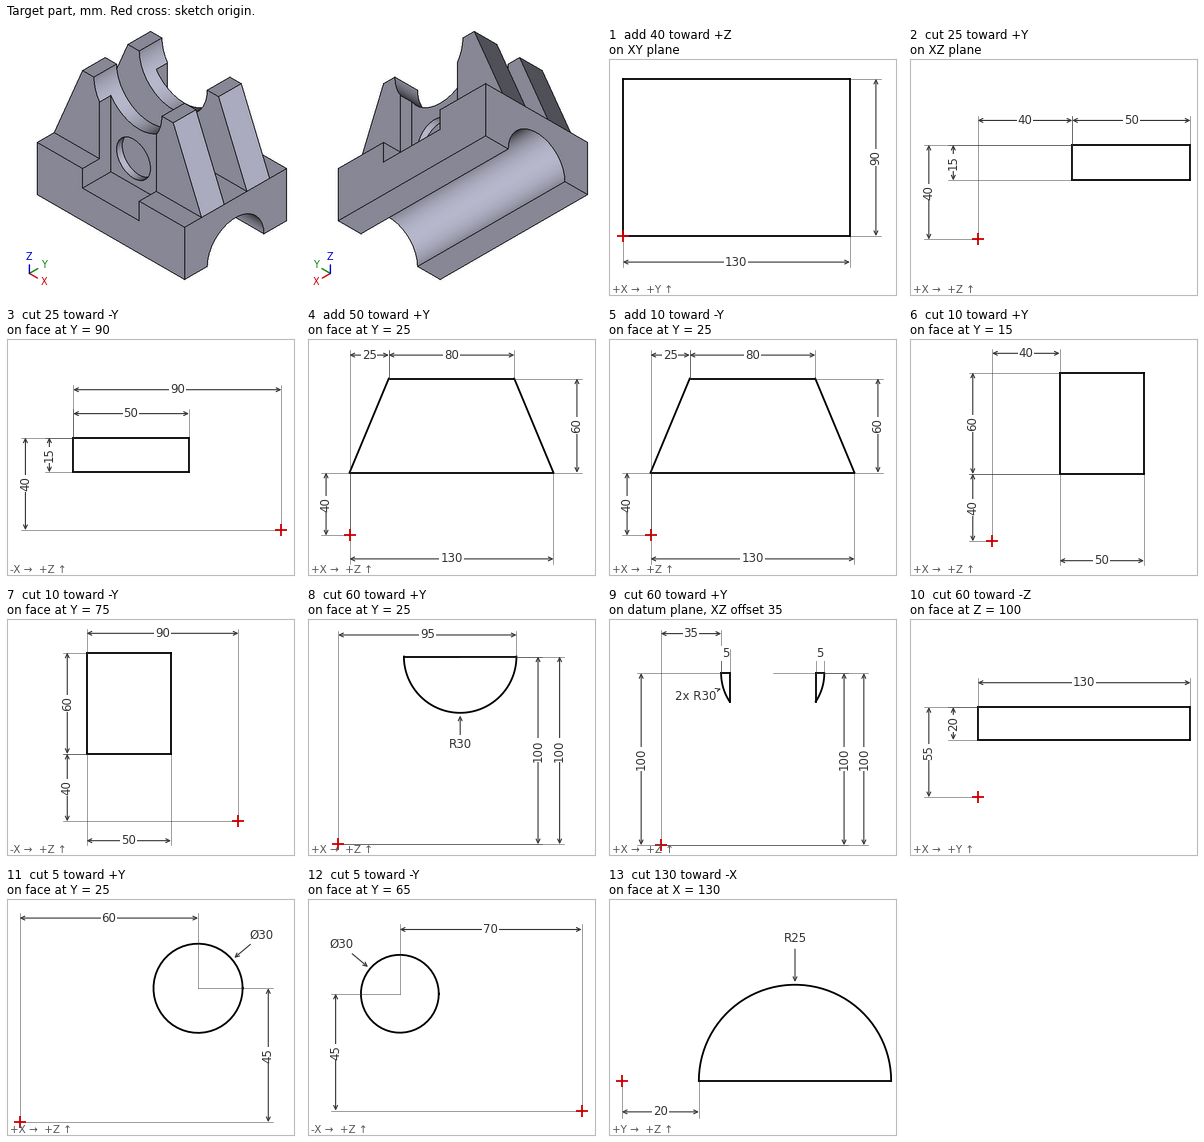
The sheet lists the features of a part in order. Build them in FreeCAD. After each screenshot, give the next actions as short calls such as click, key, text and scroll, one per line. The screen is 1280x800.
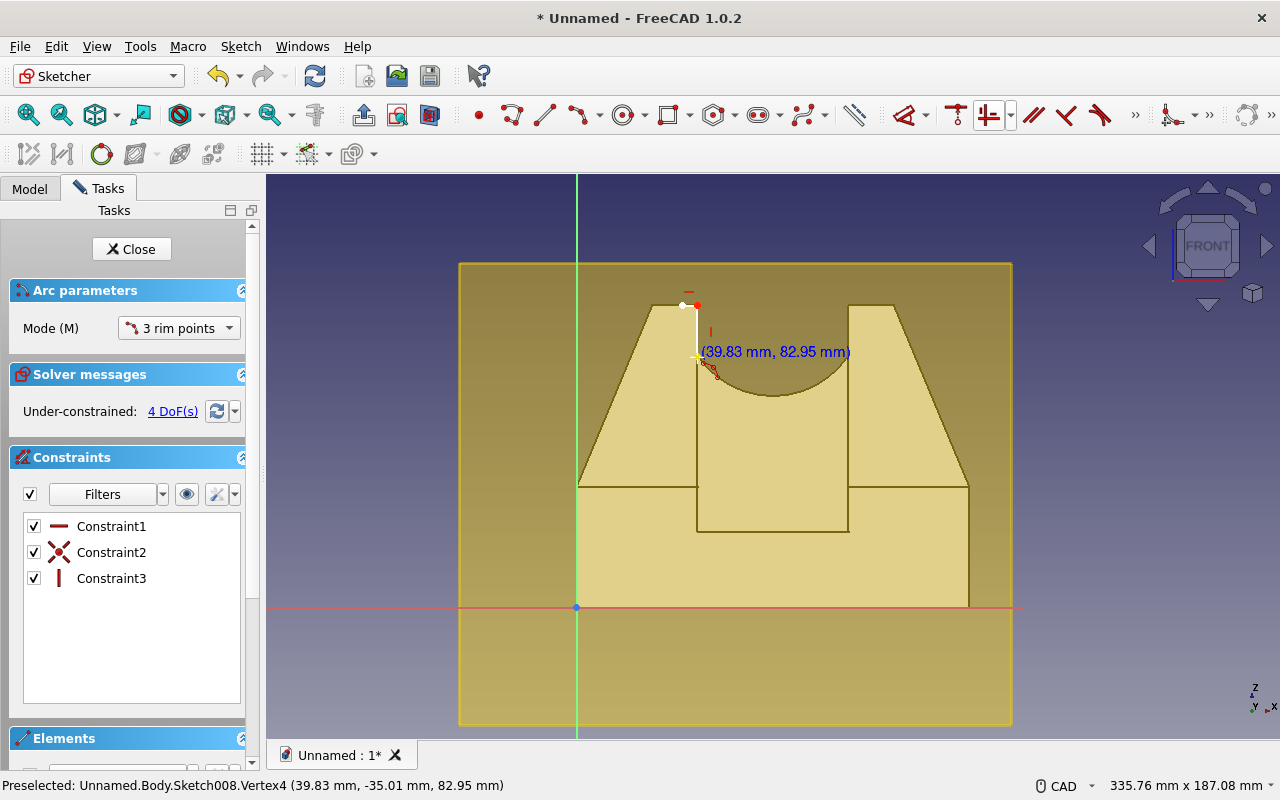
scroll(682, 305, up, 4)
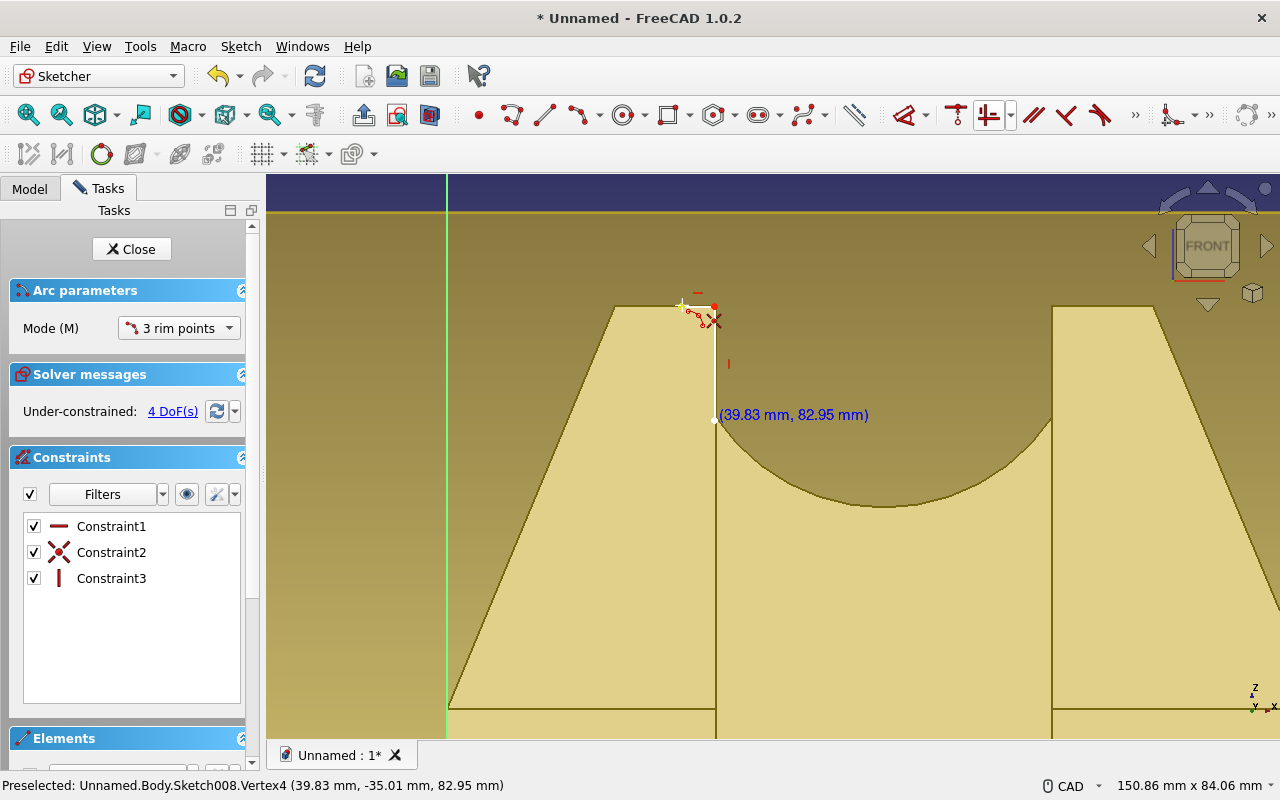
click(681, 307)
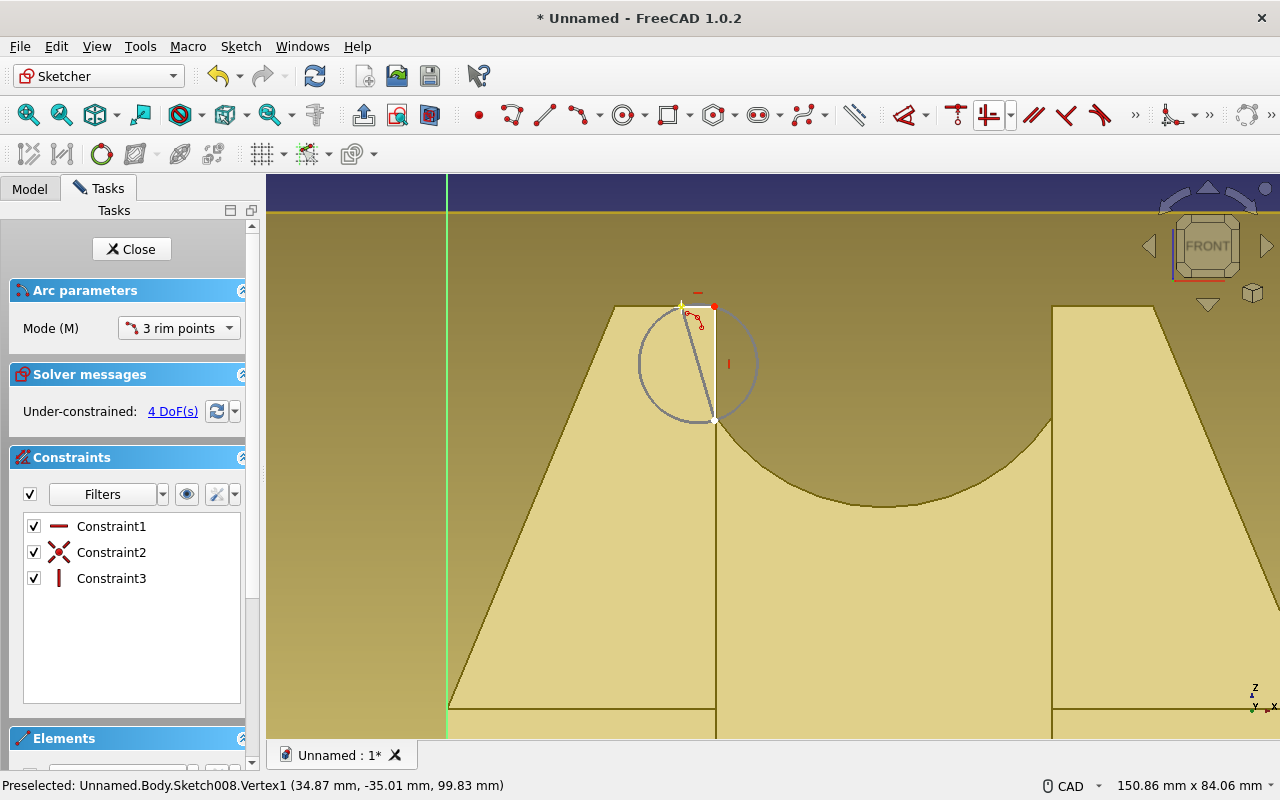
scroll(691, 364, up, 4)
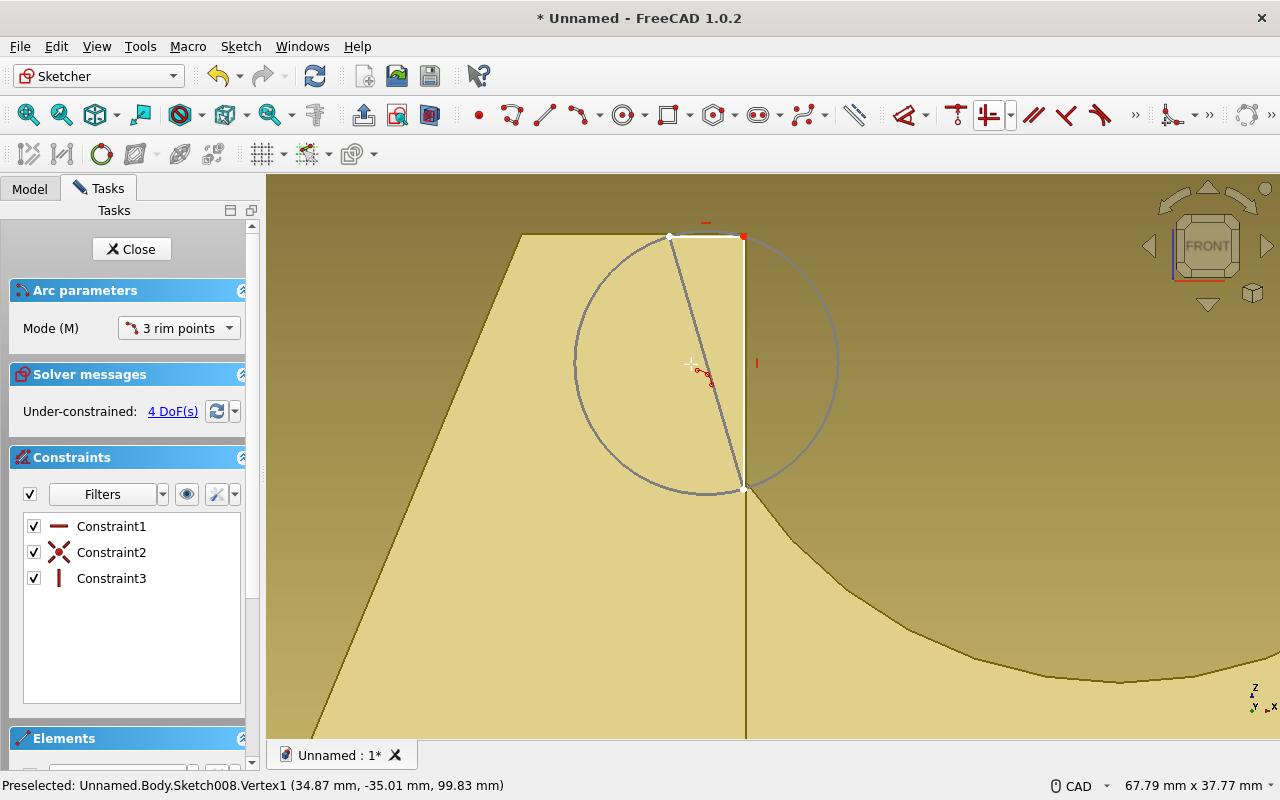
click(690, 364)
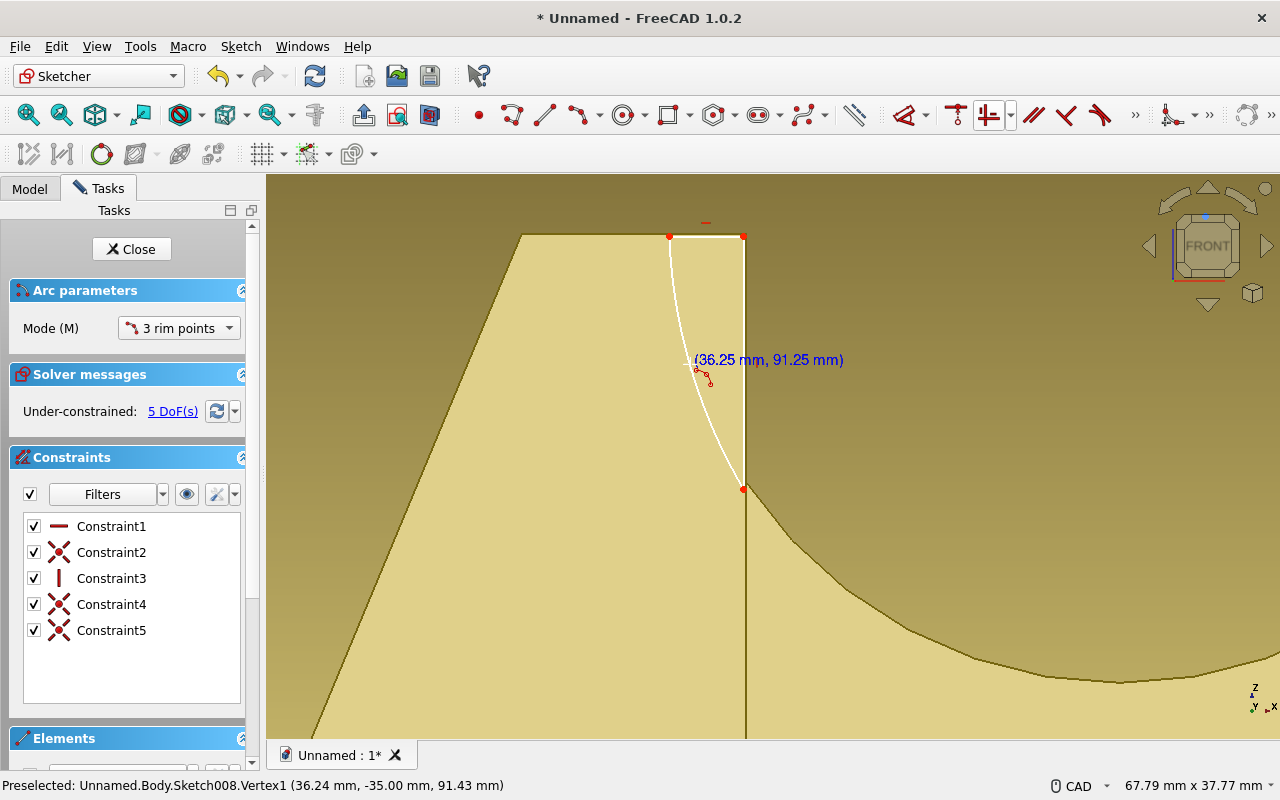
key(g)
key(m)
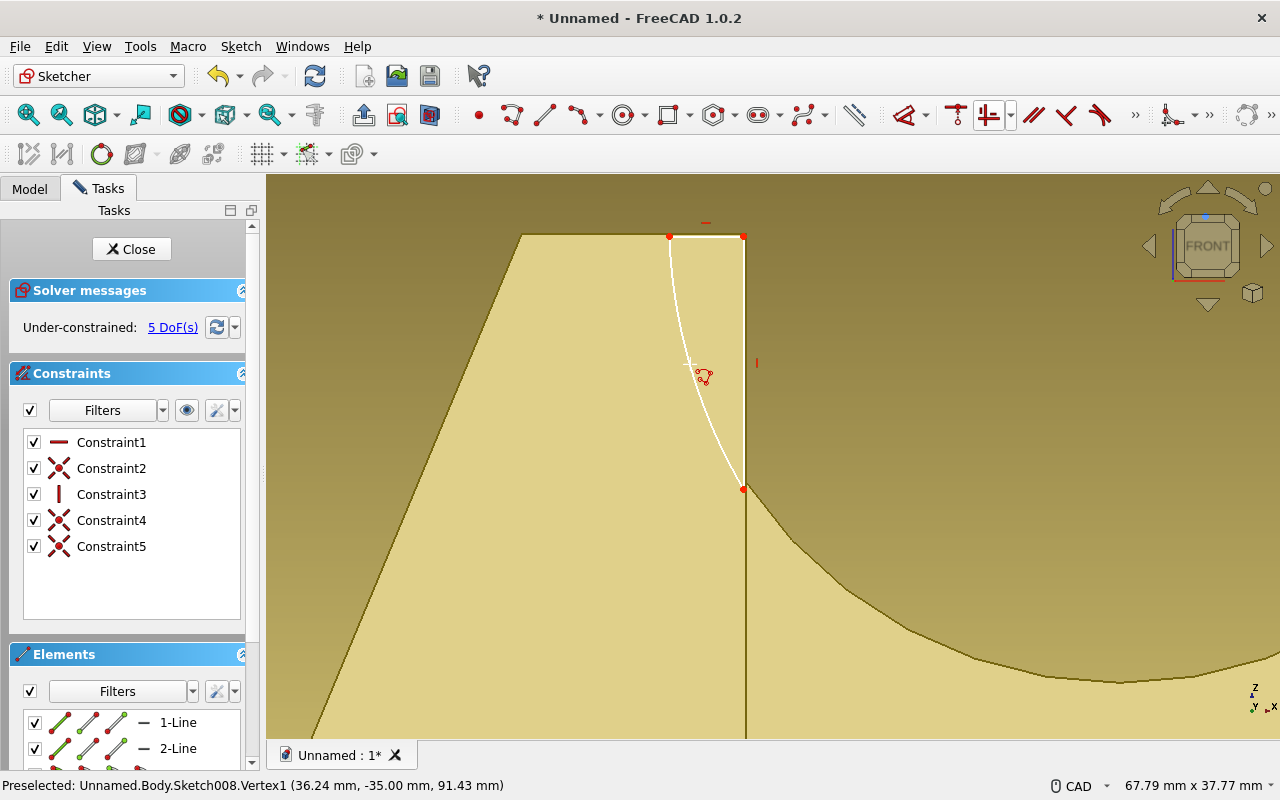
scroll(654, 284, down, 7)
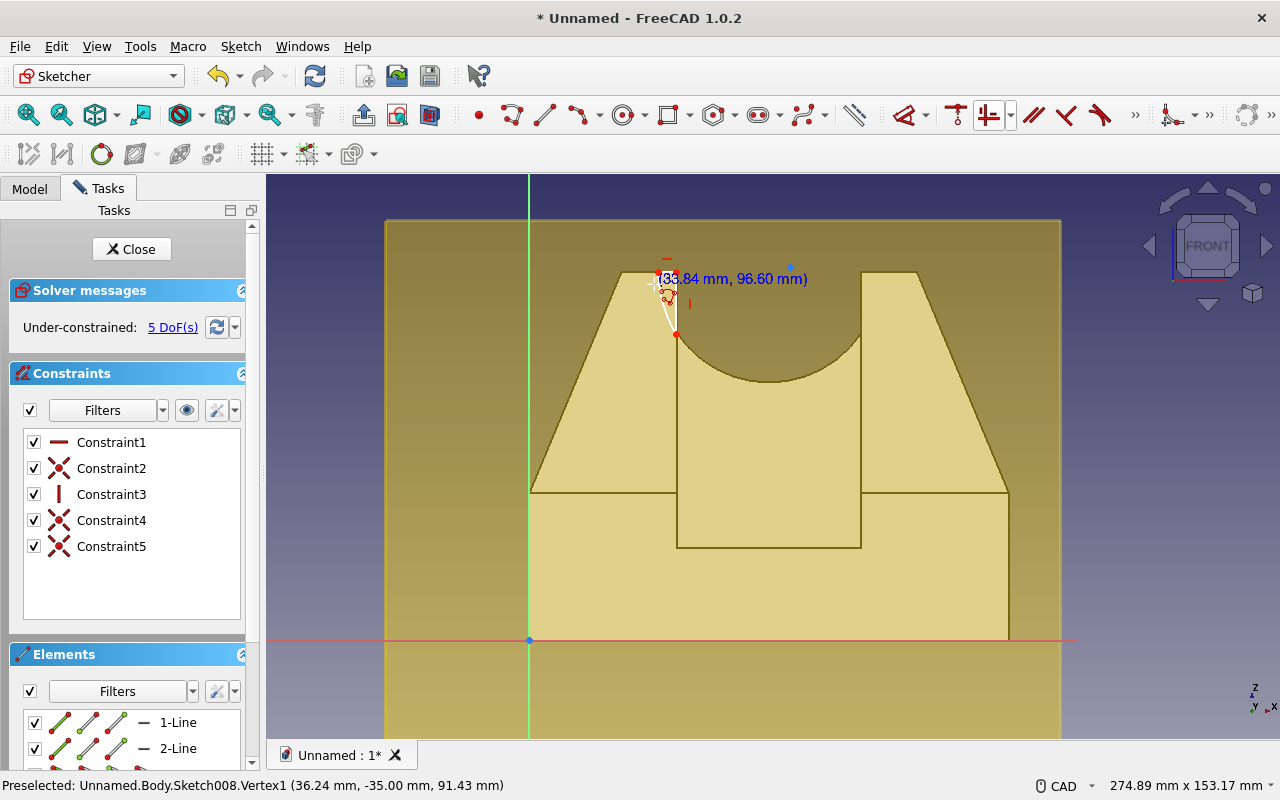
click(861, 333)
click(861, 272)
click(880, 272)
right_click(880, 272)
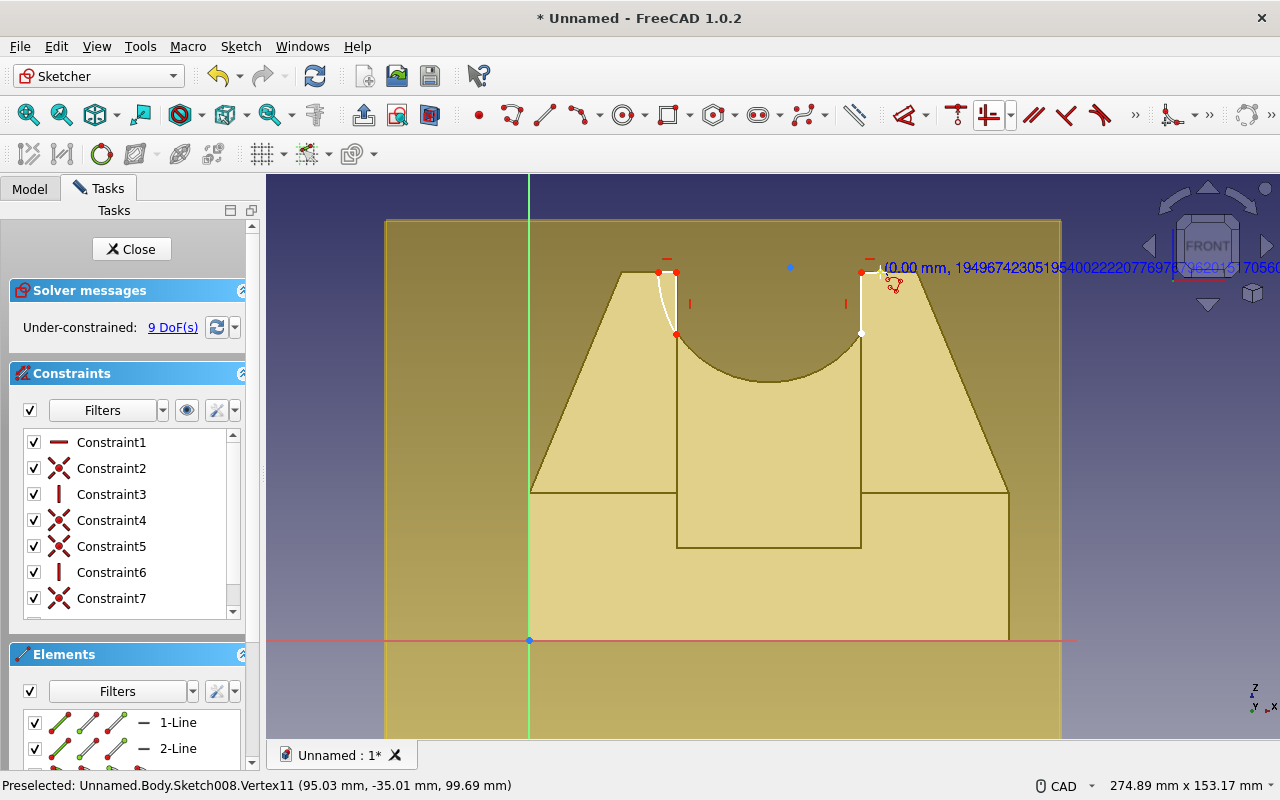
key(g)
key(3)
key(a)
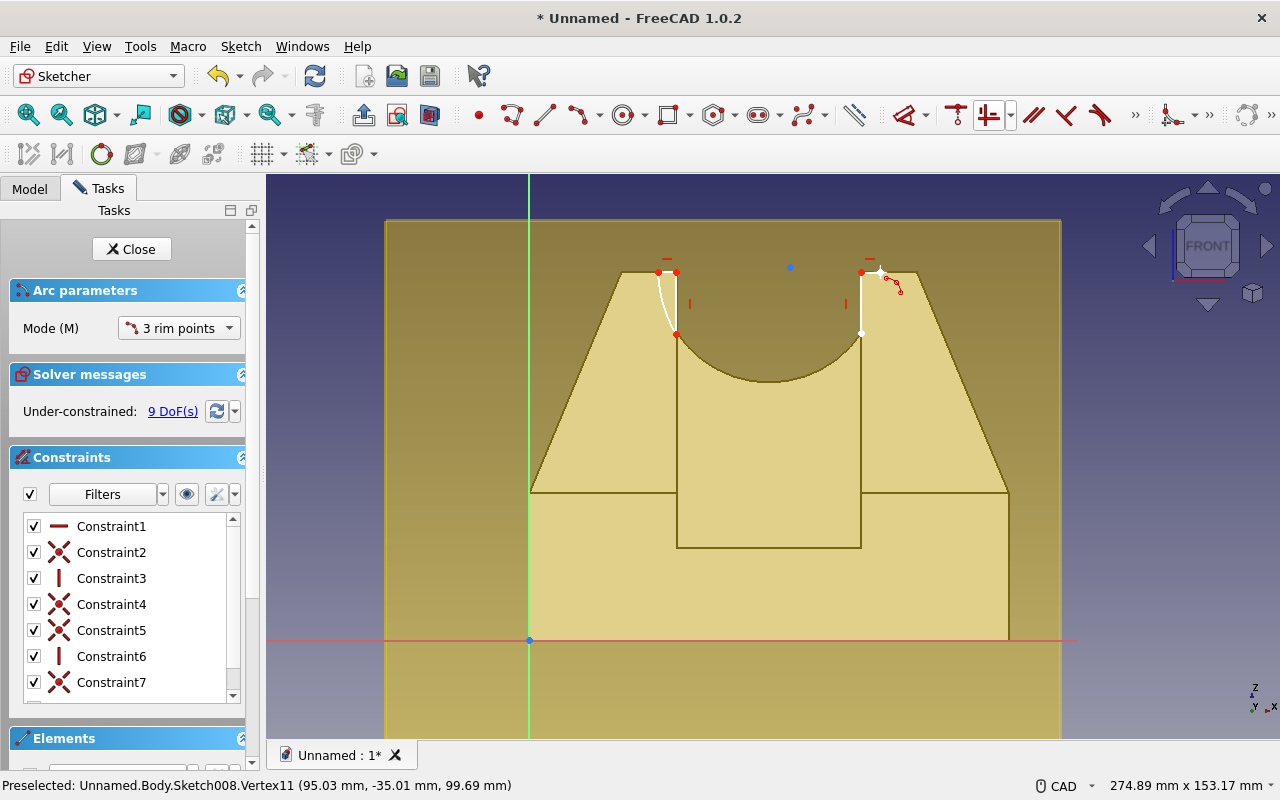
scroll(880, 272, up, 3)